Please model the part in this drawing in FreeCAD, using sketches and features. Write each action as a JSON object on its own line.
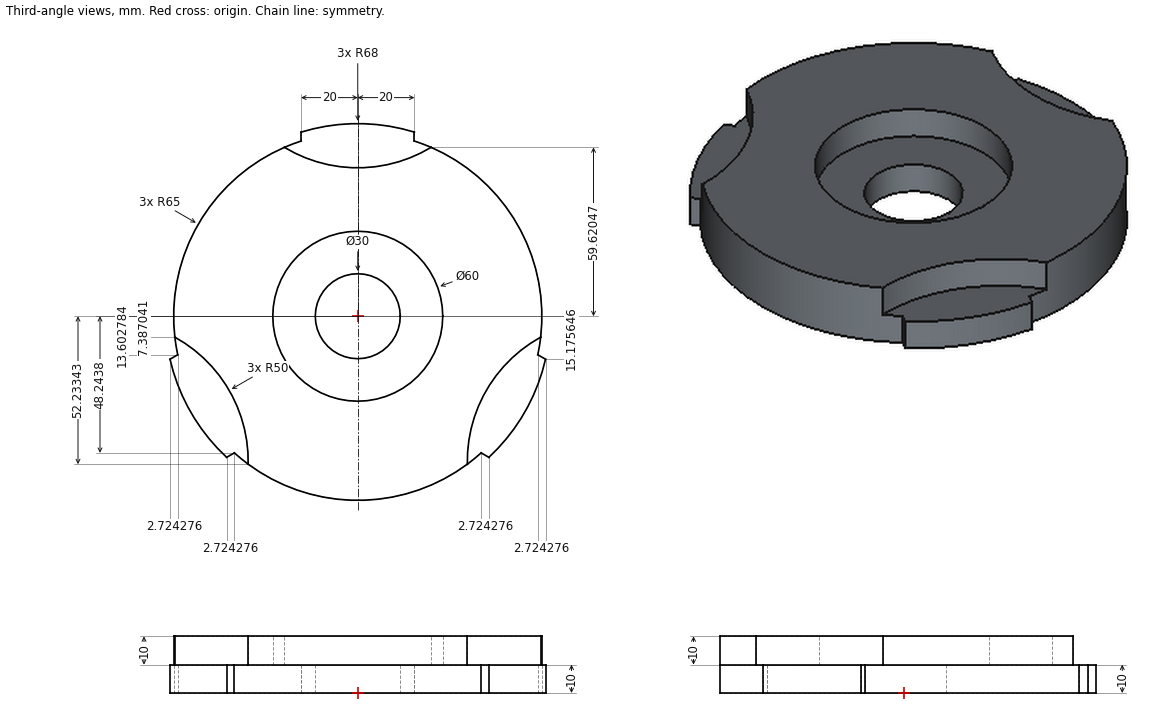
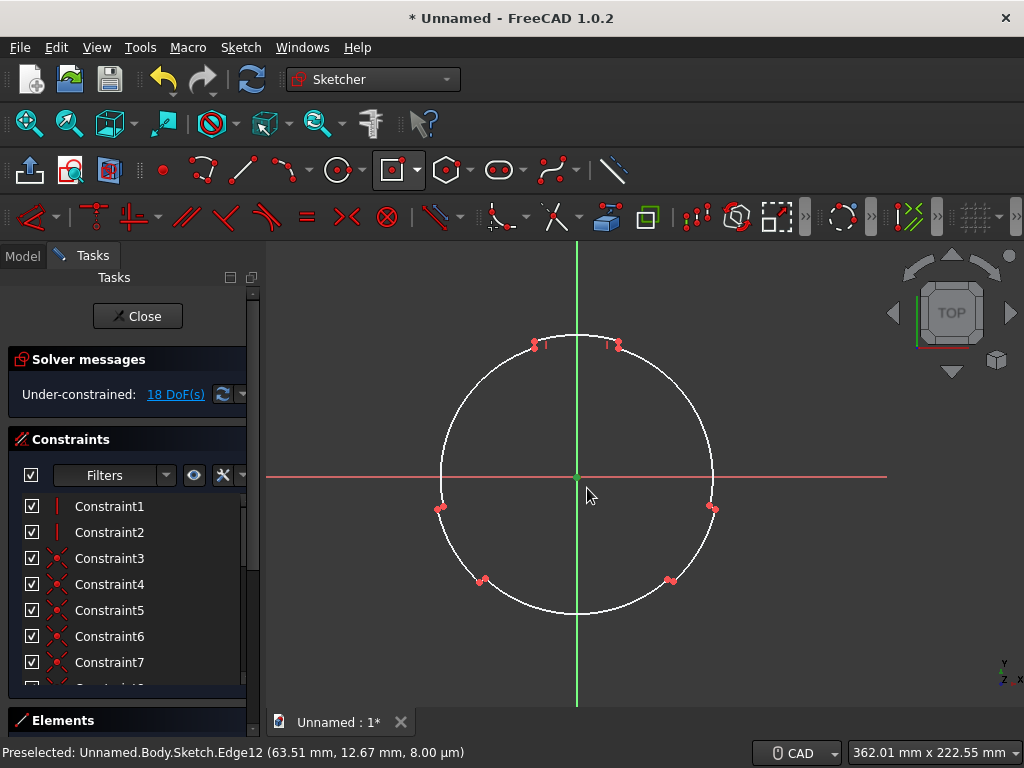
{"action": "key", "text": "c"}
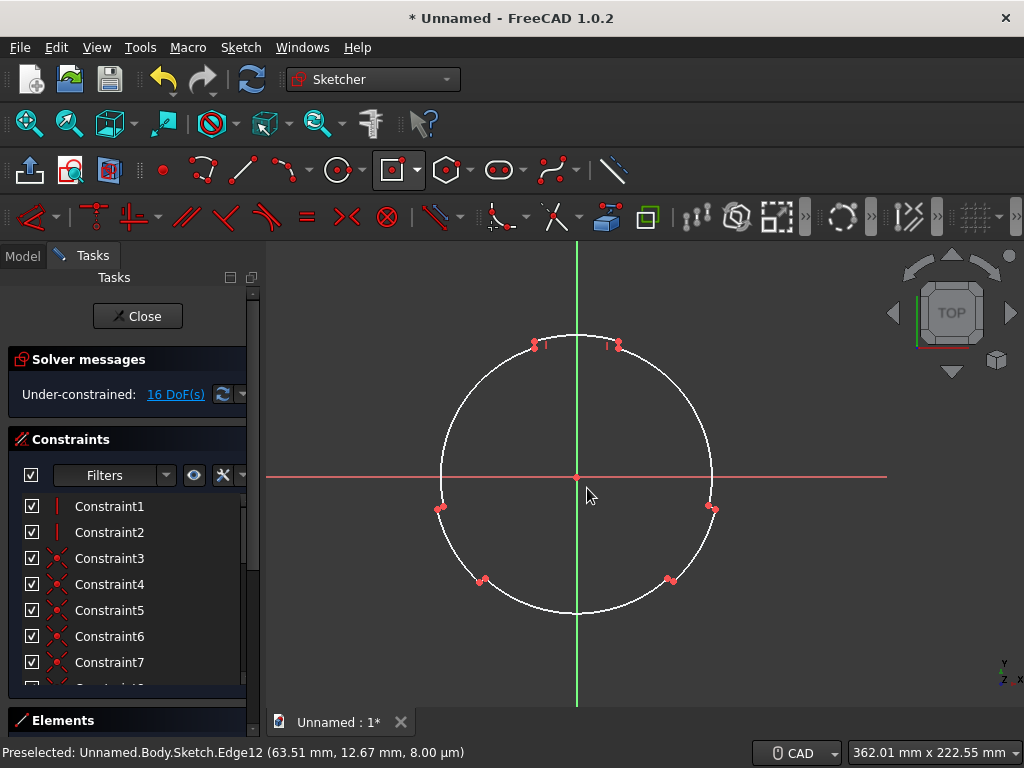
{"action": "left_click", "coordinate": [594, 336]}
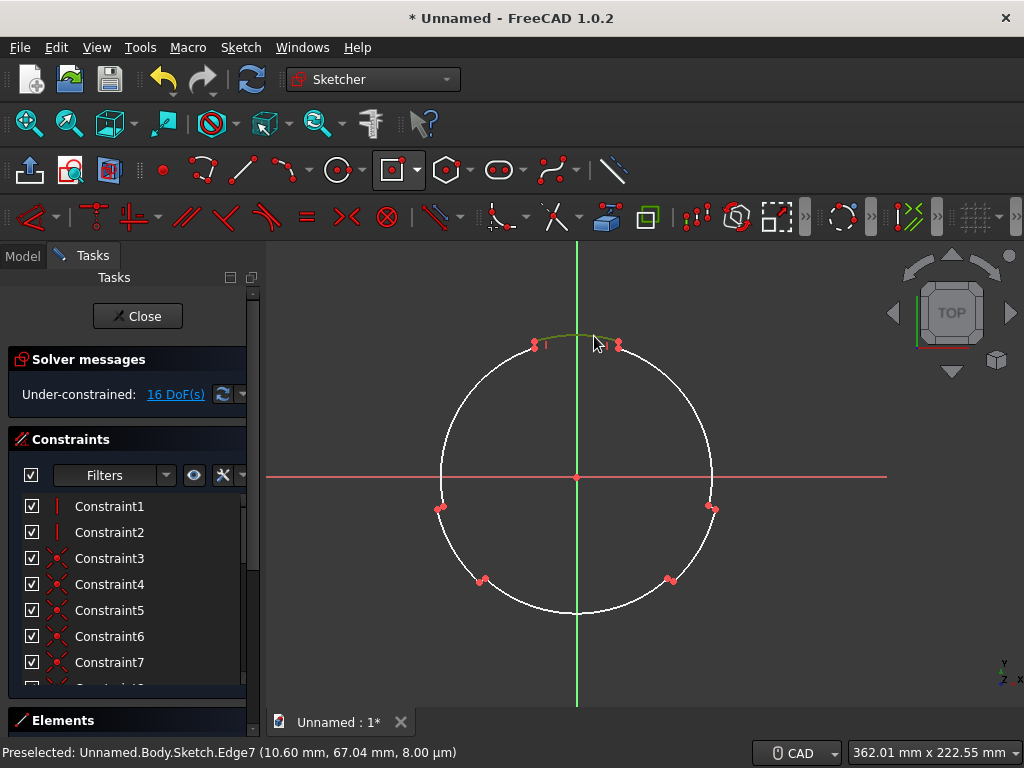
{"action": "left_click", "coordinate": [445, 534]}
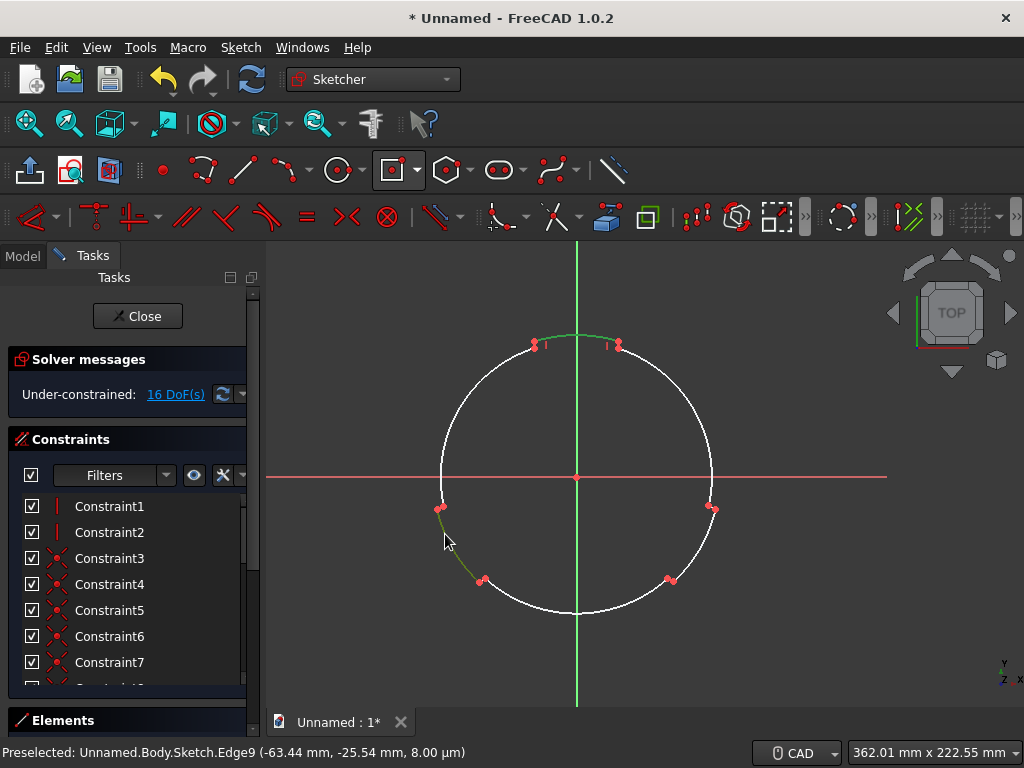
{"action": "left_click", "coordinate": [691, 563]}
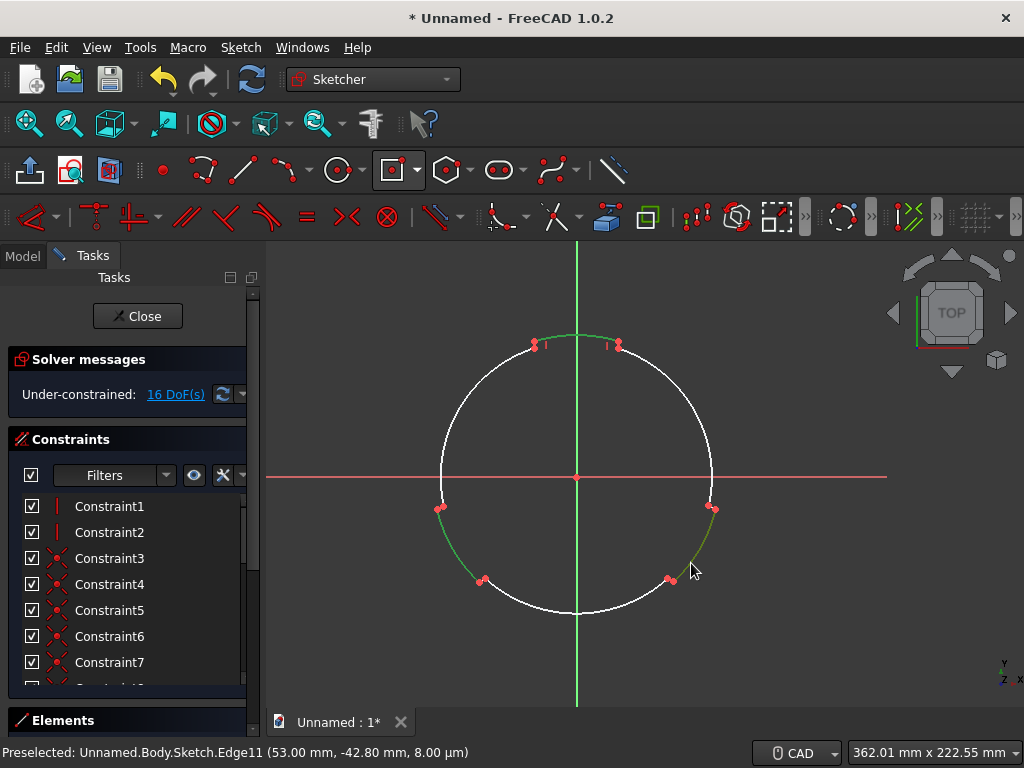
{"action": "left_click", "coordinate": [308, 218]}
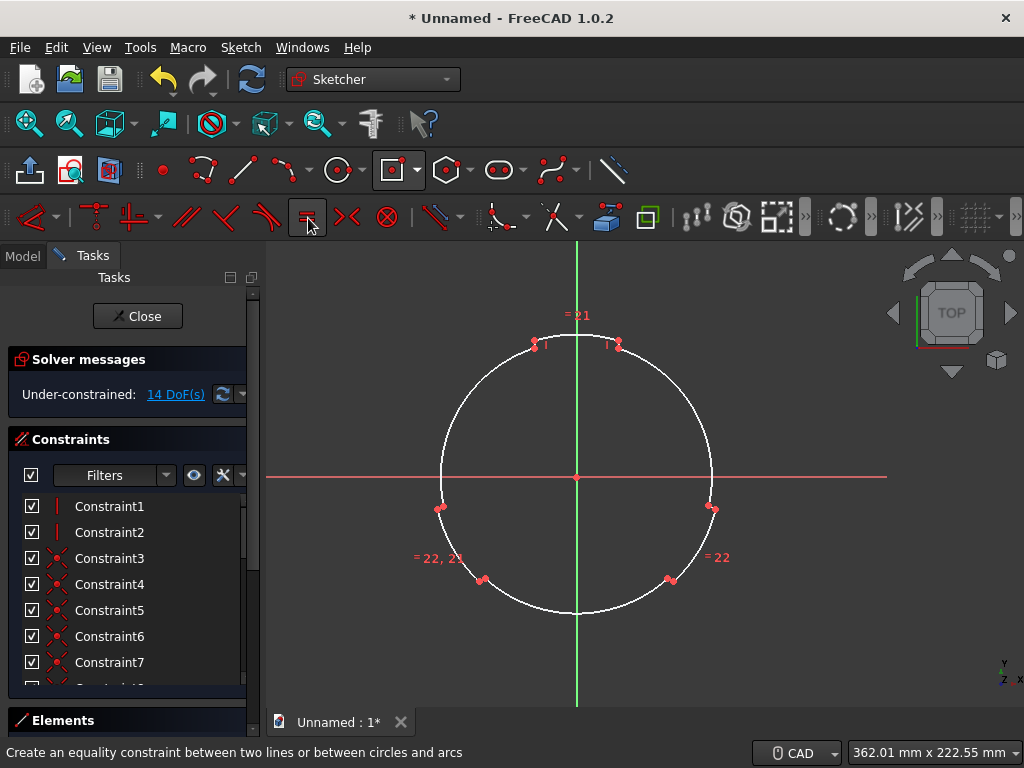
{"action": "left_click", "coordinate": [483, 378]}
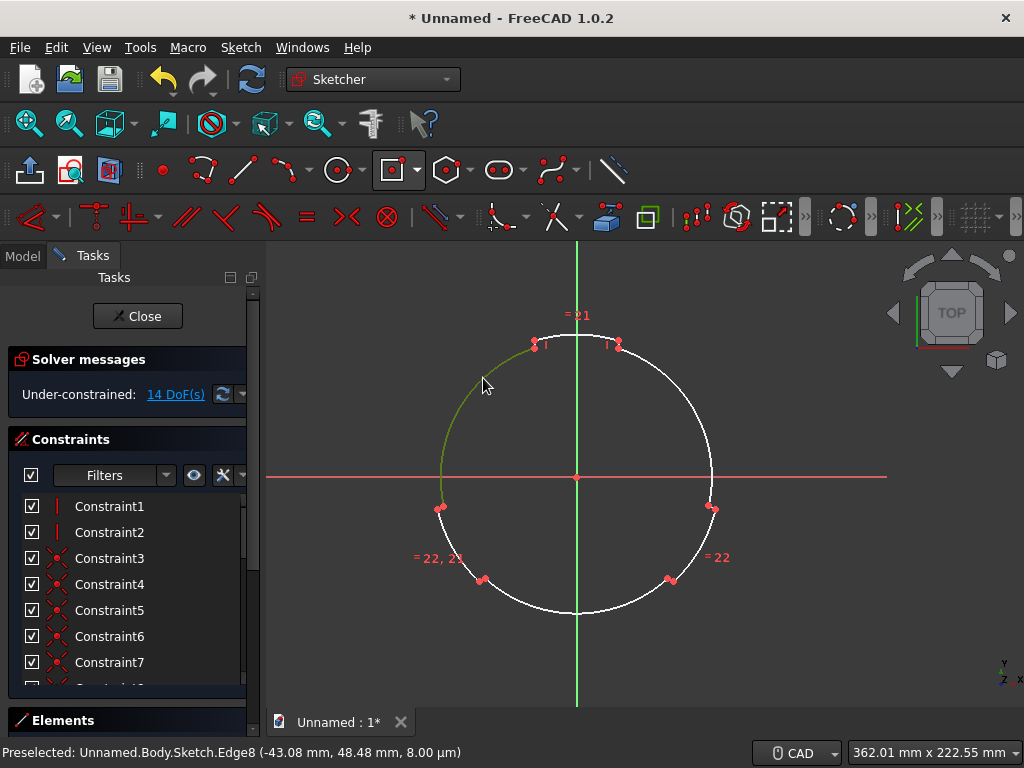
{"action": "left_click", "coordinate": [537, 608]}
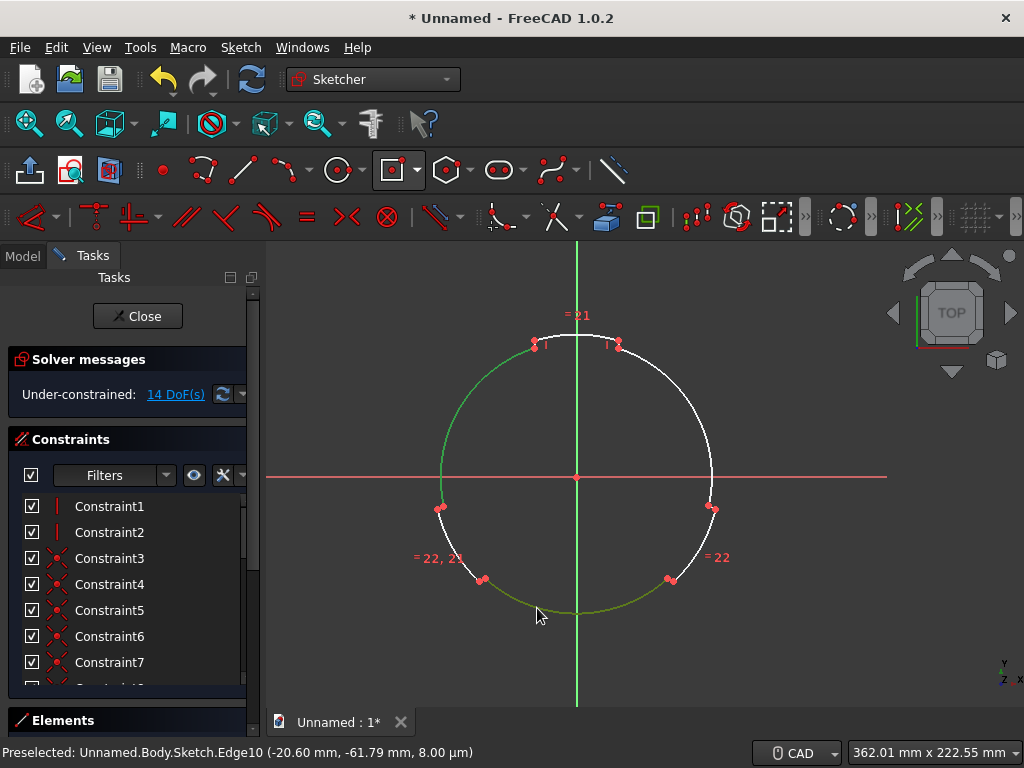
{"action": "left_click", "coordinate": [708, 447]}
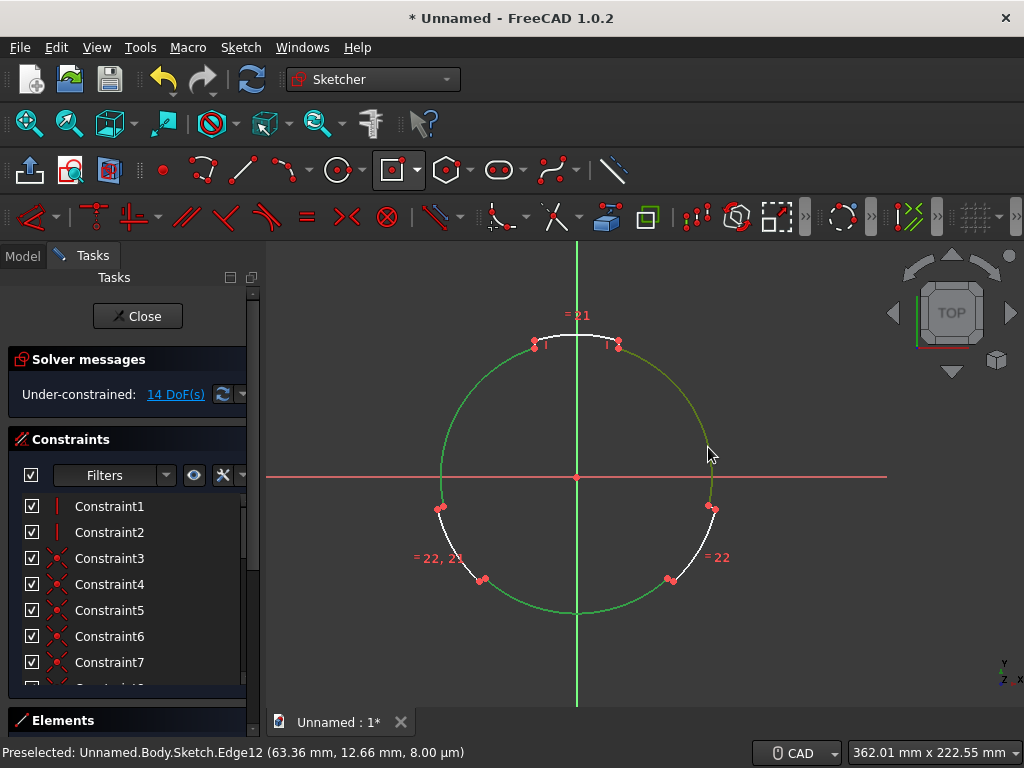
{"action": "left_click", "coordinate": [308, 218]}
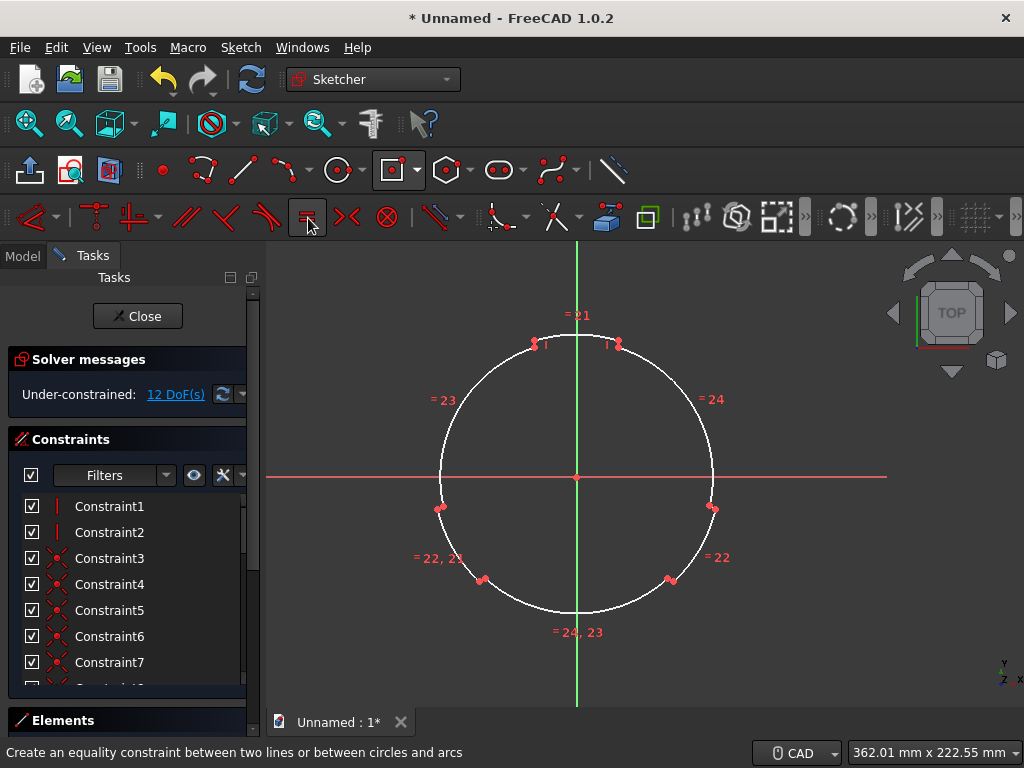
{"action": "left_click", "coordinate": [594, 336]}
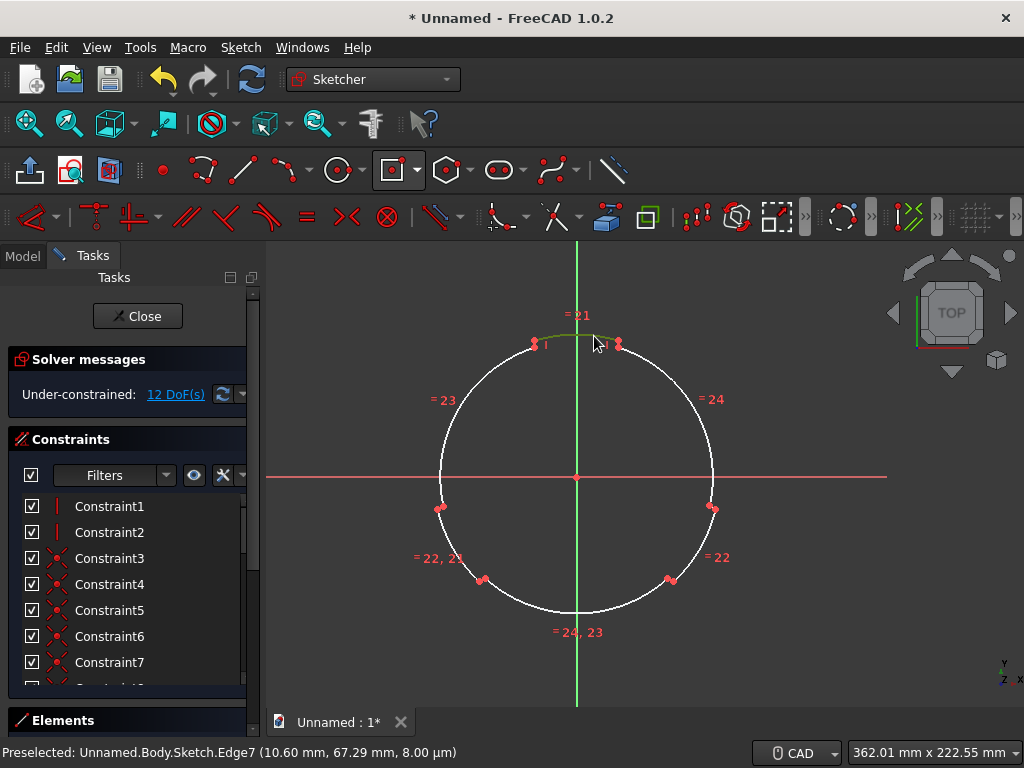
{"action": "key", "text": "k r"}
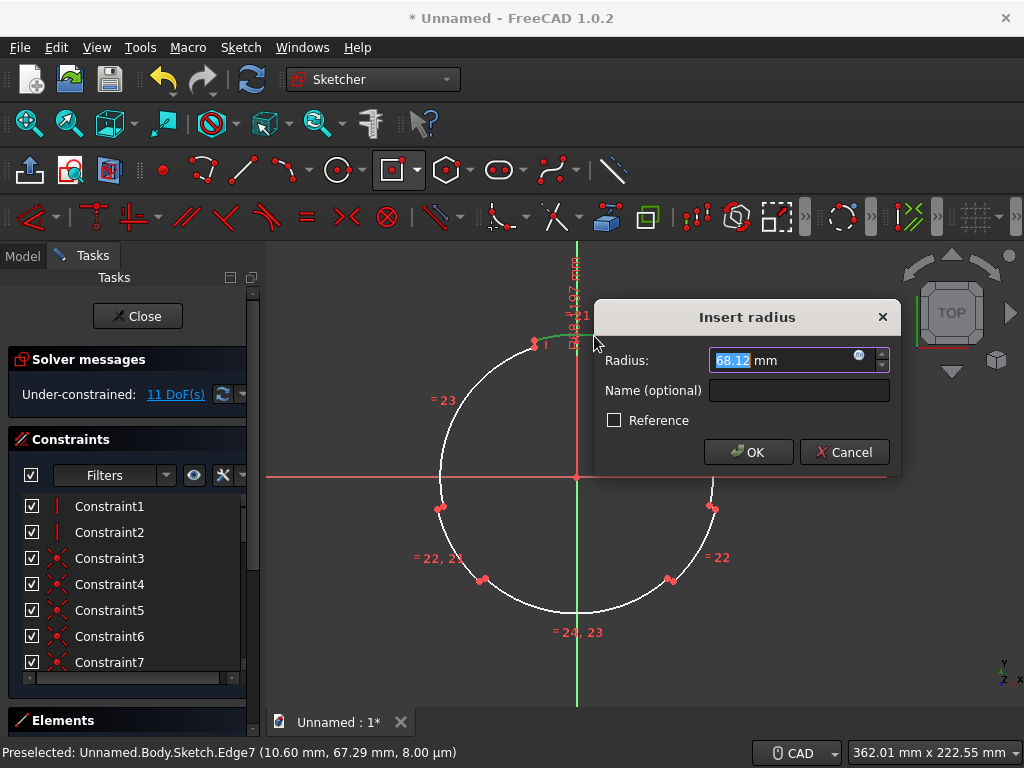
{"action": "type", "text": "68"}
{"action": "key", "text": "Return"}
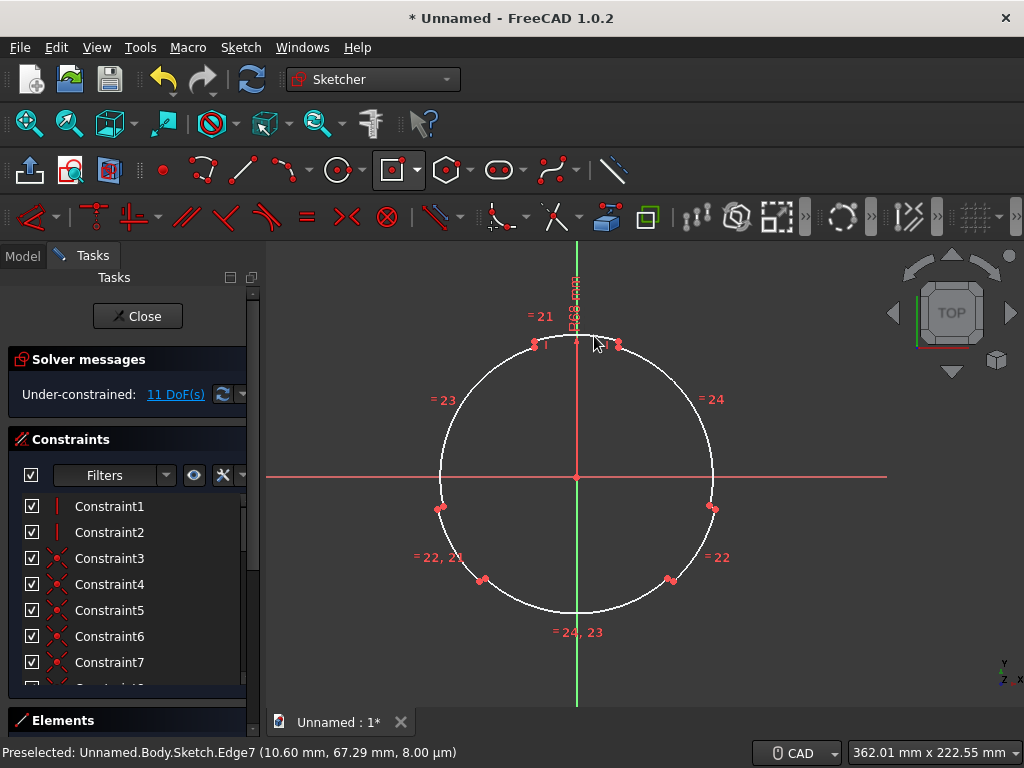
{"action": "left_click", "coordinate": [483, 378]}